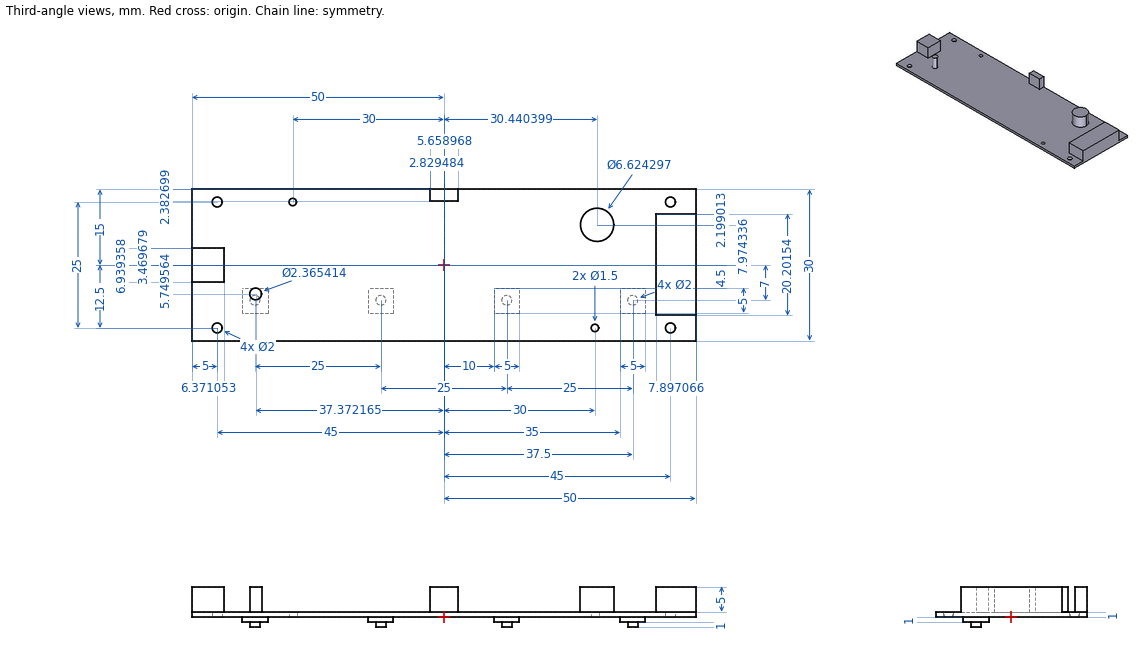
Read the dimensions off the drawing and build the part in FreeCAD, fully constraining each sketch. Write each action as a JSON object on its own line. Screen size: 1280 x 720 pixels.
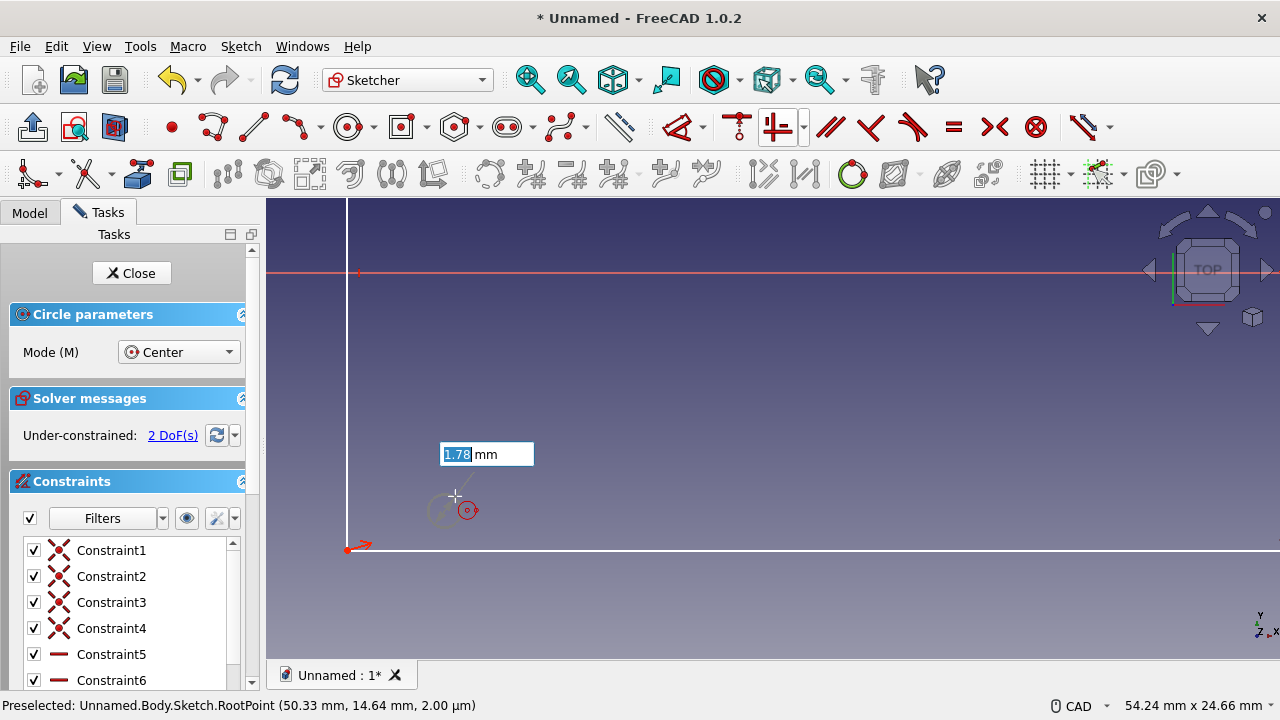
{"action": "left_click", "coordinate": [456, 493]}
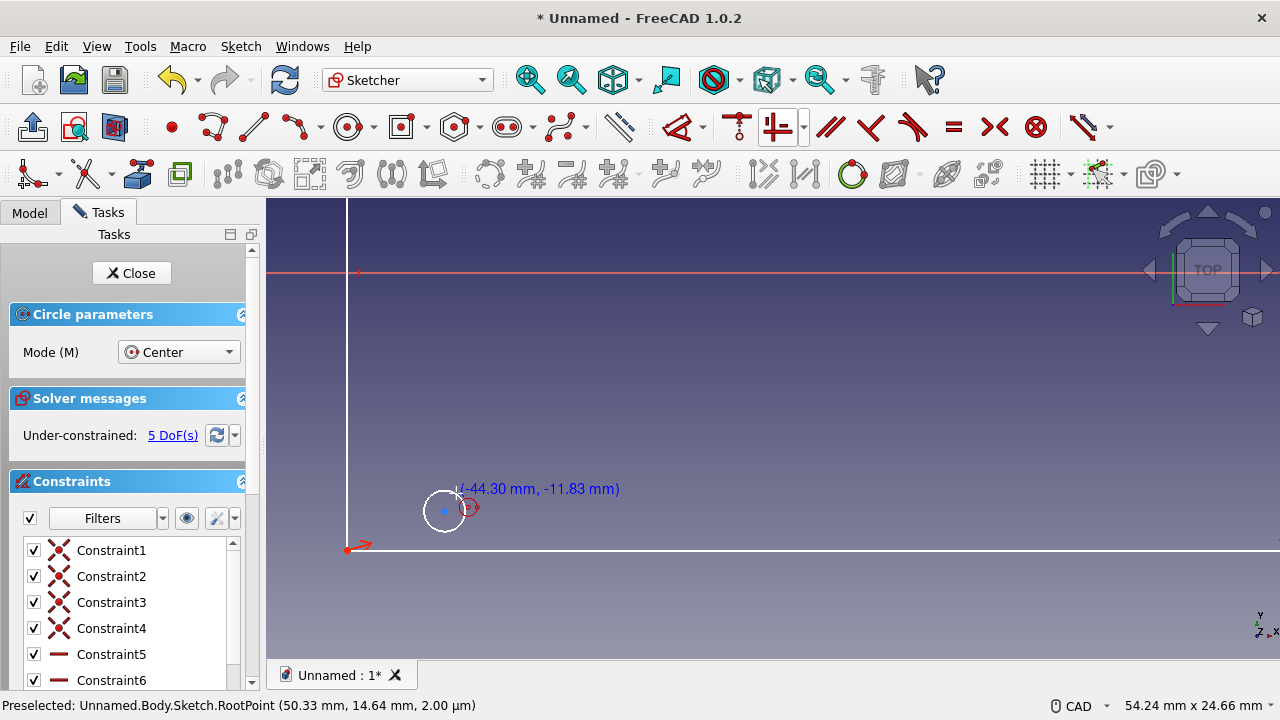
{"action": "scroll", "coordinate": [455, 496], "scroll_direction": "down", "scroll_amount": 6}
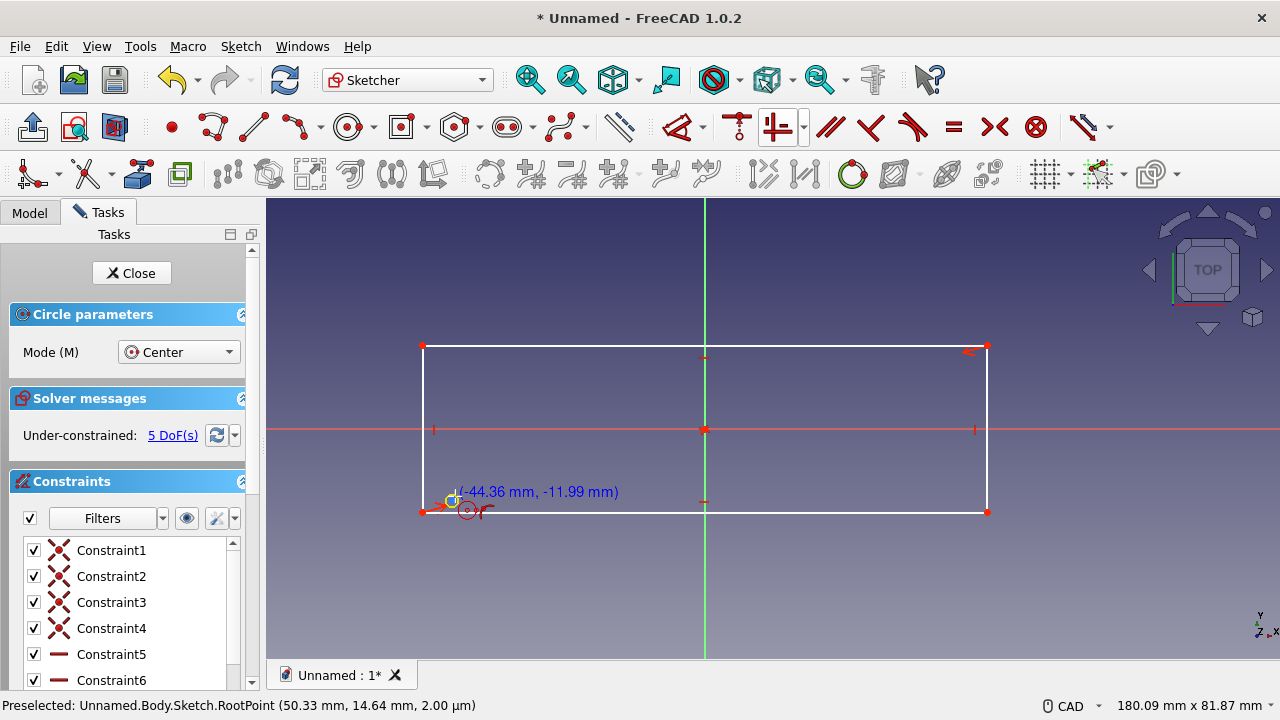
{"action": "scroll", "coordinate": [958, 500], "scroll_direction": "up", "scroll_amount": 7}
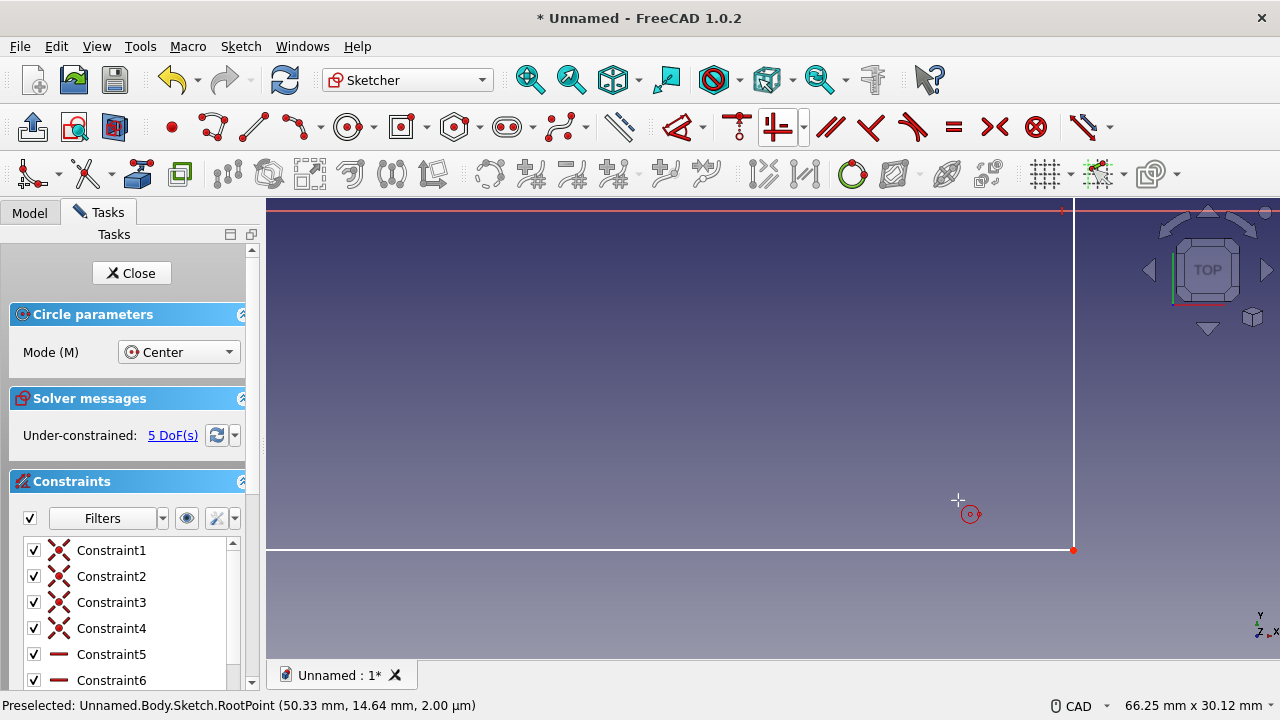
{"action": "scroll", "coordinate": [958, 500], "scroll_direction": "down", "scroll_amount": 7}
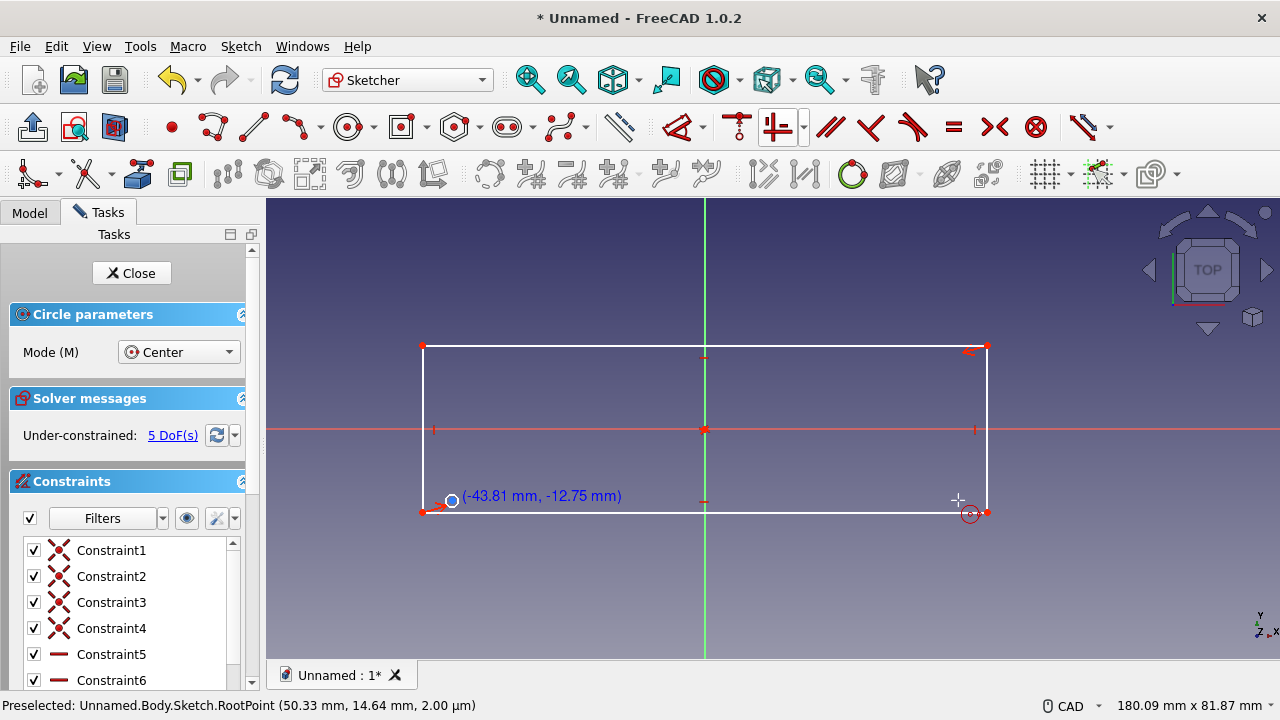
{"action": "left_click", "coordinate": [958, 500]}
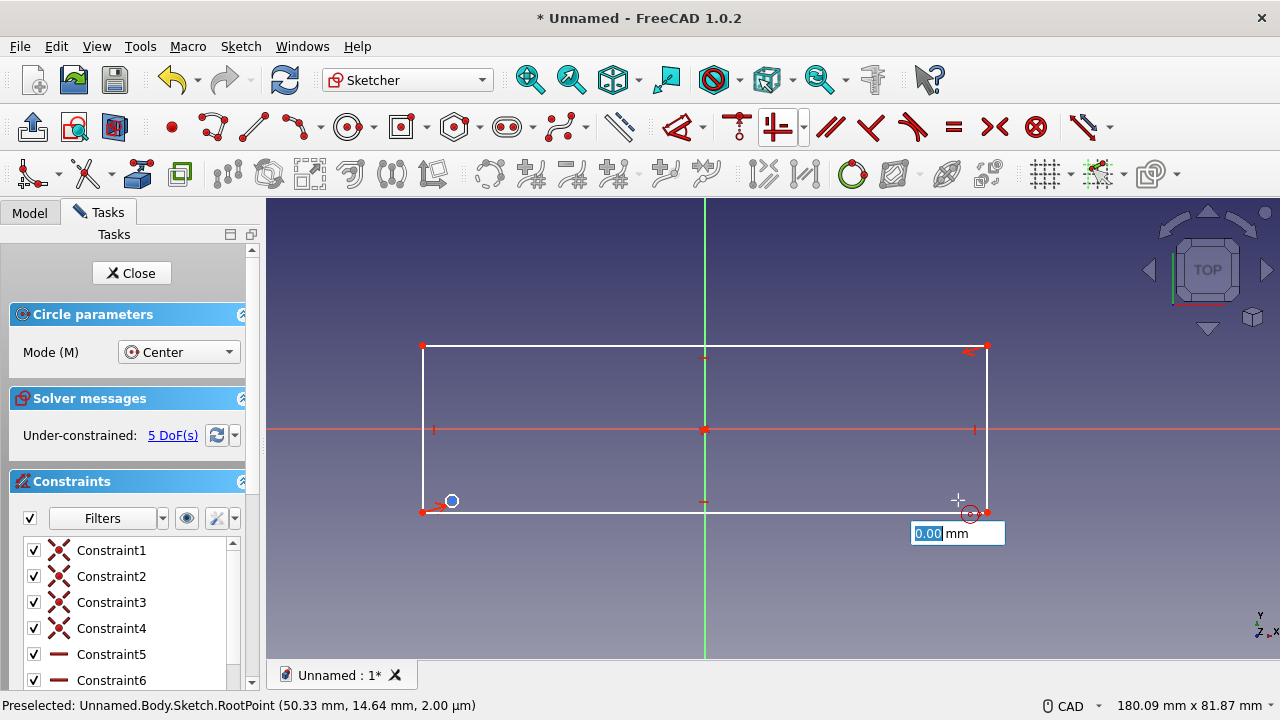
{"action": "scroll", "coordinate": [962, 496], "scroll_direction": "up", "scroll_amount": 6}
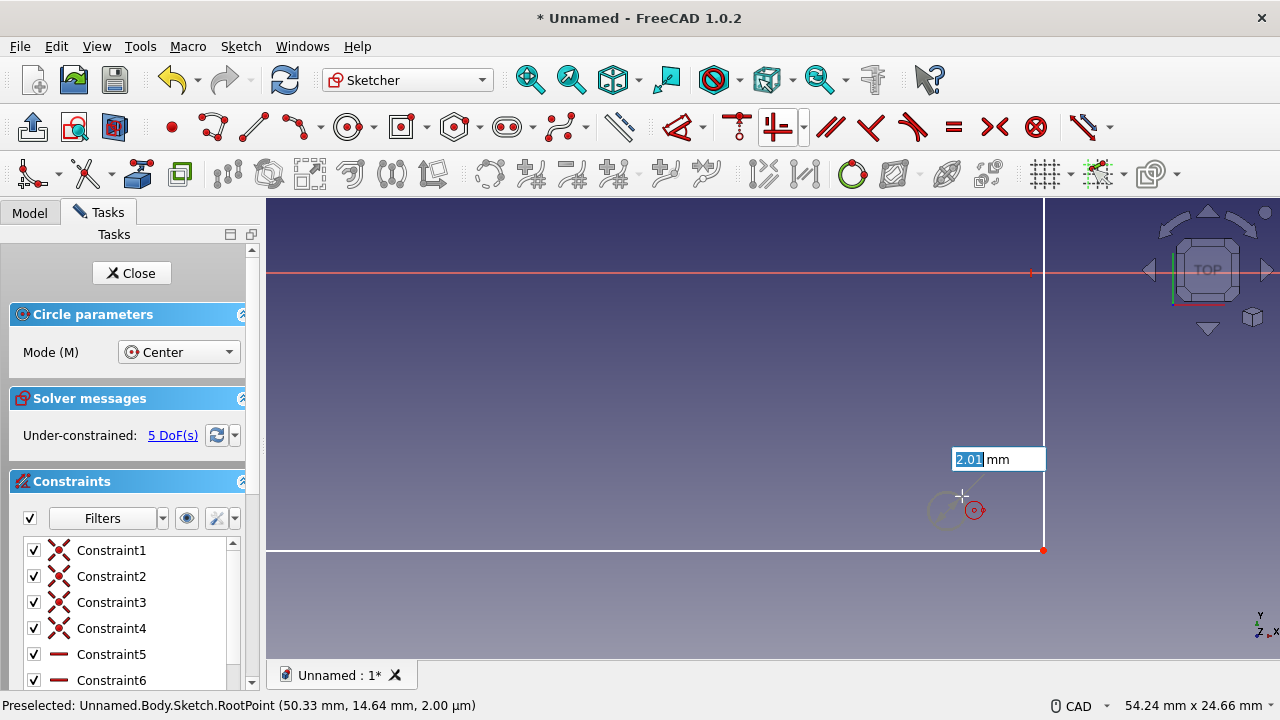
{"action": "left_click", "coordinate": [961, 493]}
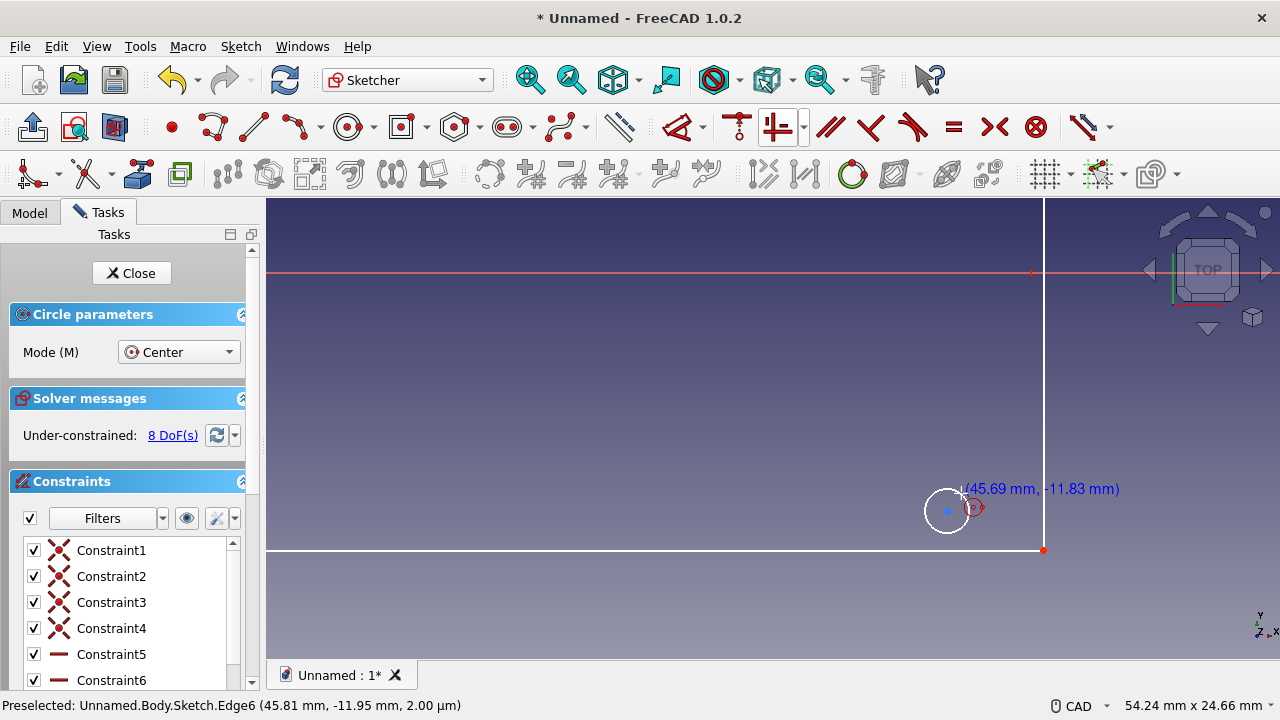
{"action": "scroll", "coordinate": [962, 496], "scroll_direction": "down", "scroll_amount": 6}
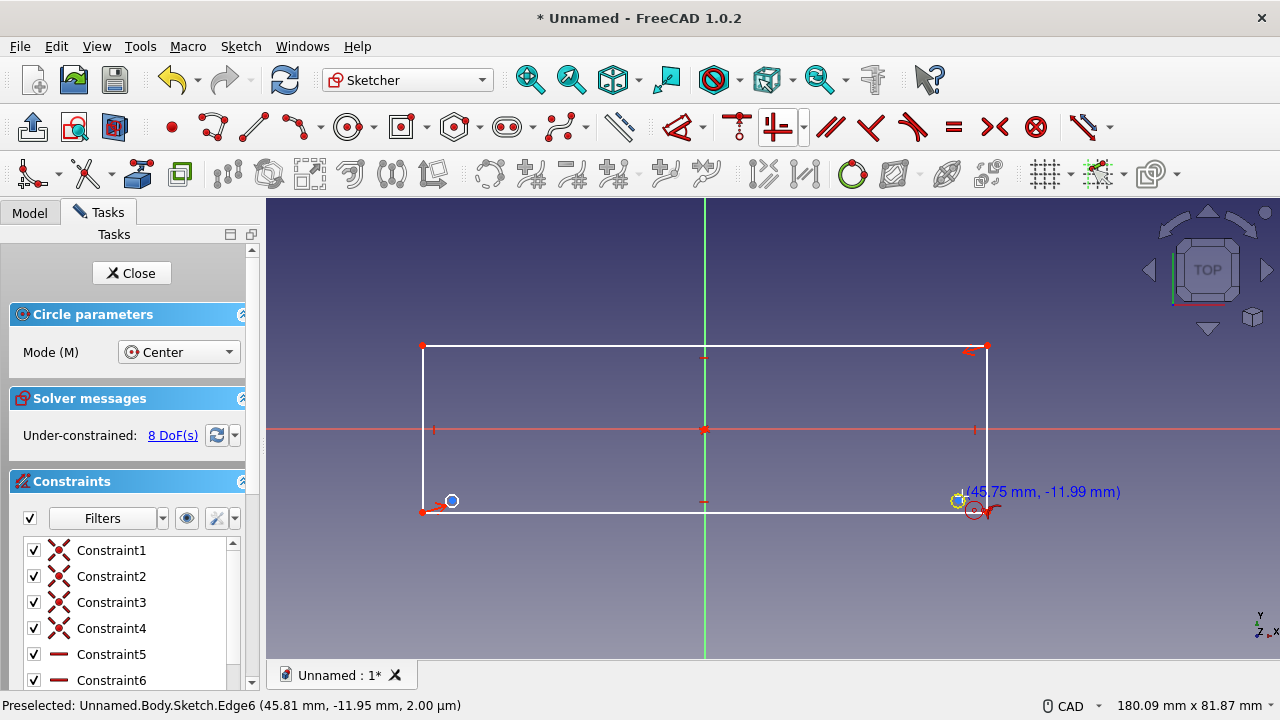
{"action": "scroll", "coordinate": [452, 359], "scroll_direction": "up", "scroll_amount": 7}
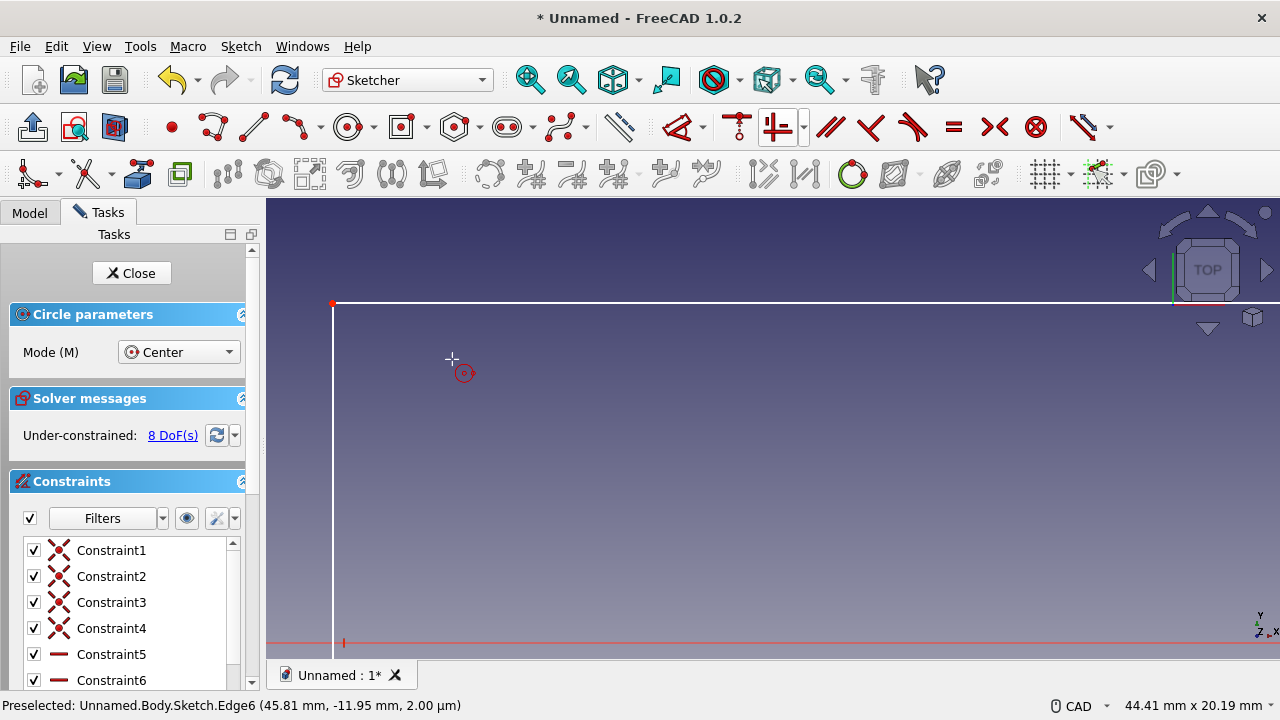
{"action": "scroll", "coordinate": [452, 358], "scroll_direction": "down", "scroll_amount": 7}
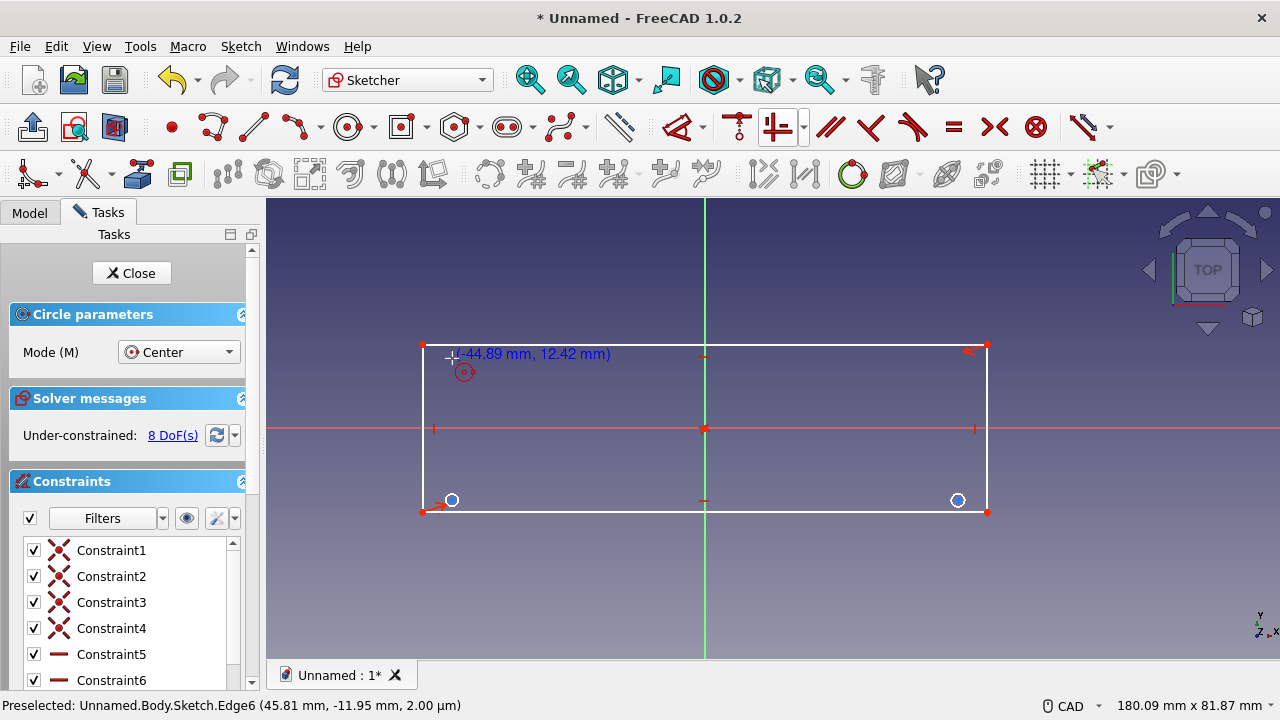
{"action": "left_click", "coordinate": [452, 358]}